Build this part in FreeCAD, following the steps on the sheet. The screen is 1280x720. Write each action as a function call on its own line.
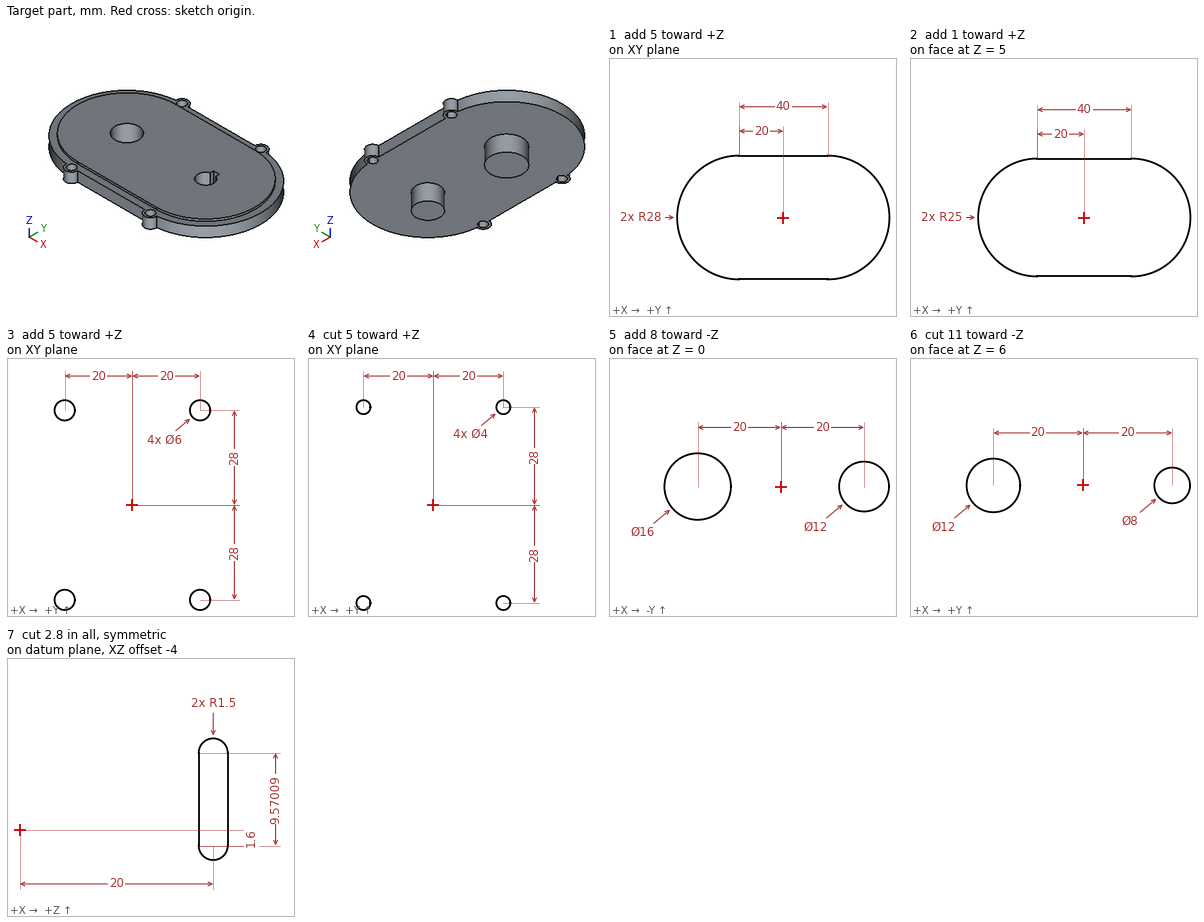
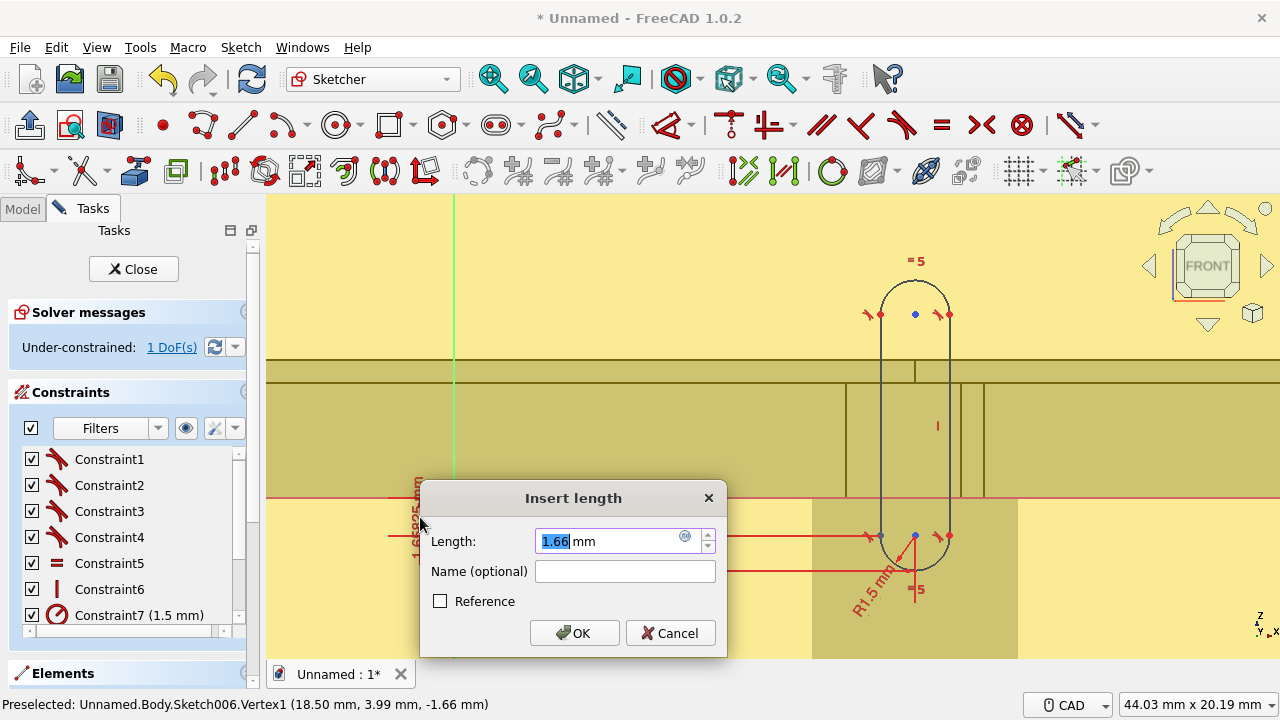
text(1.6)
key(Return)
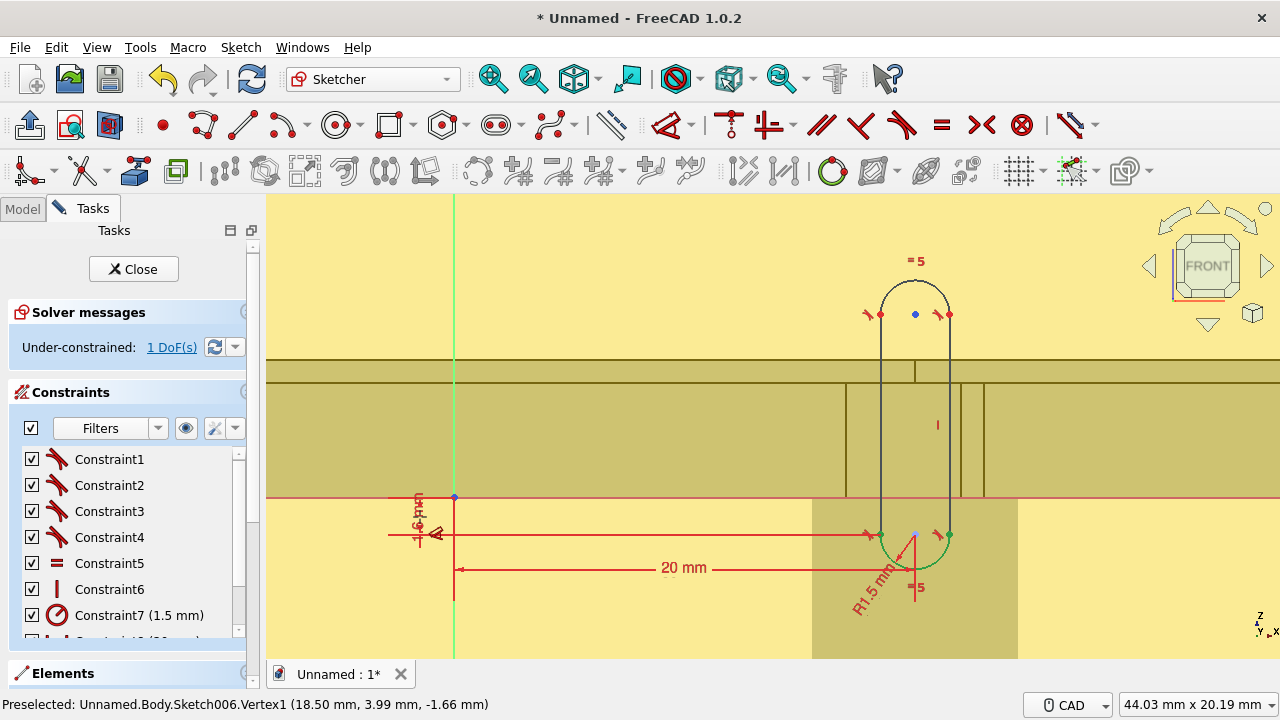
click(881, 469)
click(915, 425)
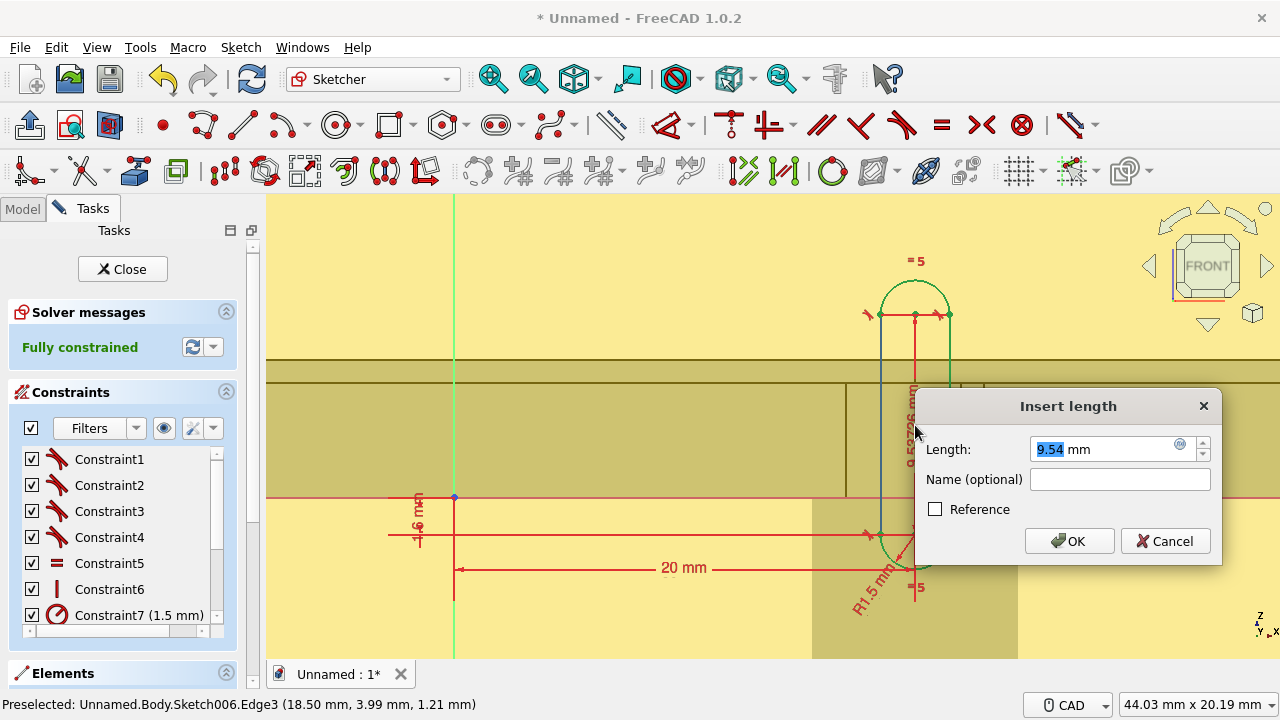
text(9.57009)
key(Return)
key(Escape)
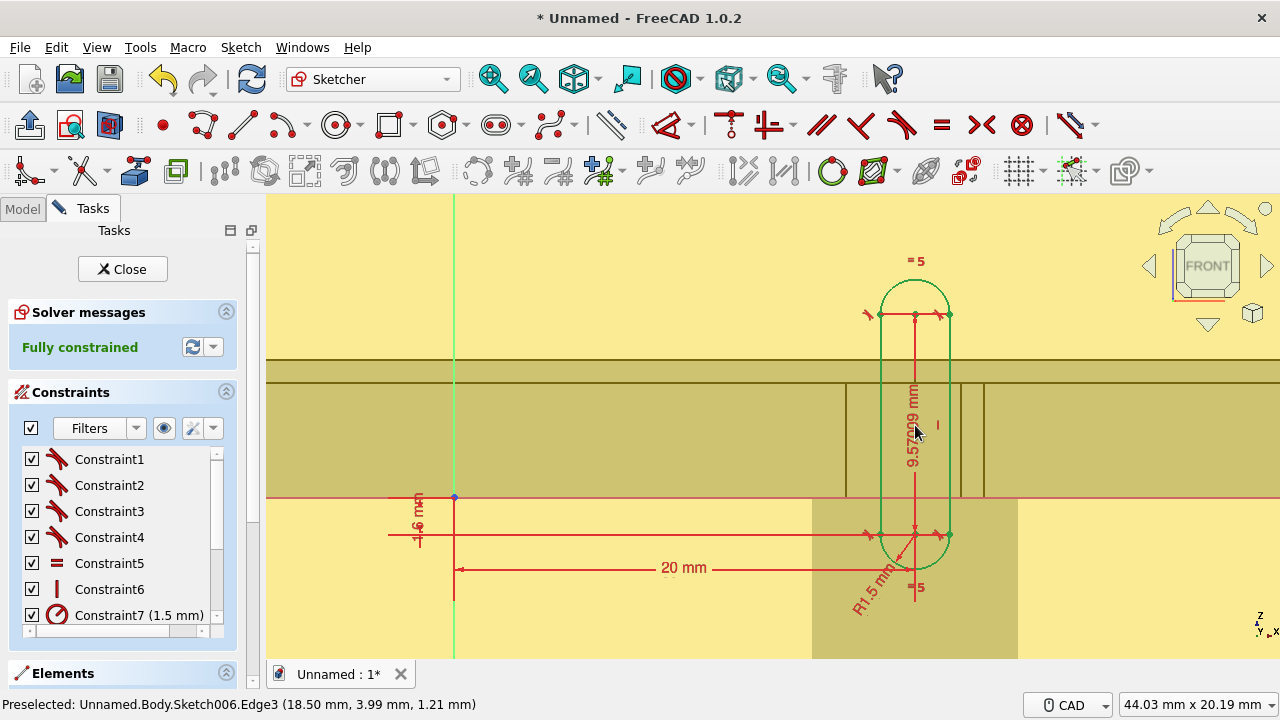
click(123, 269)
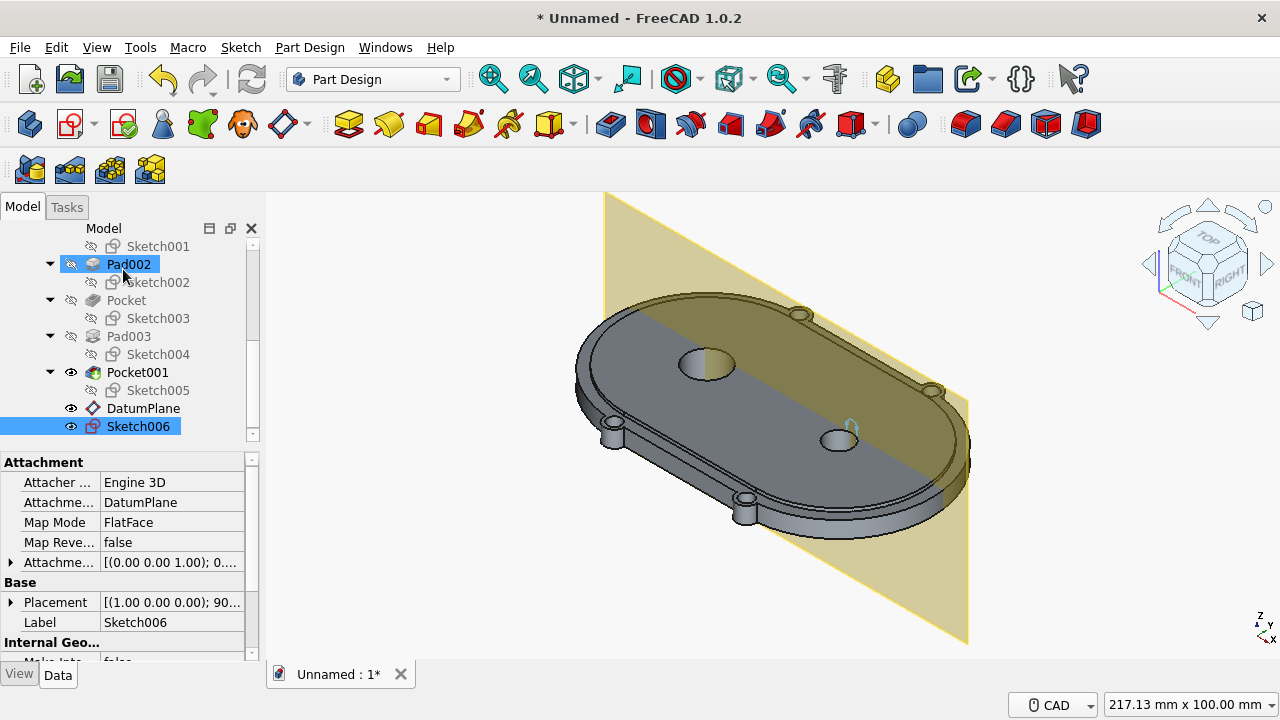
click(612, 124)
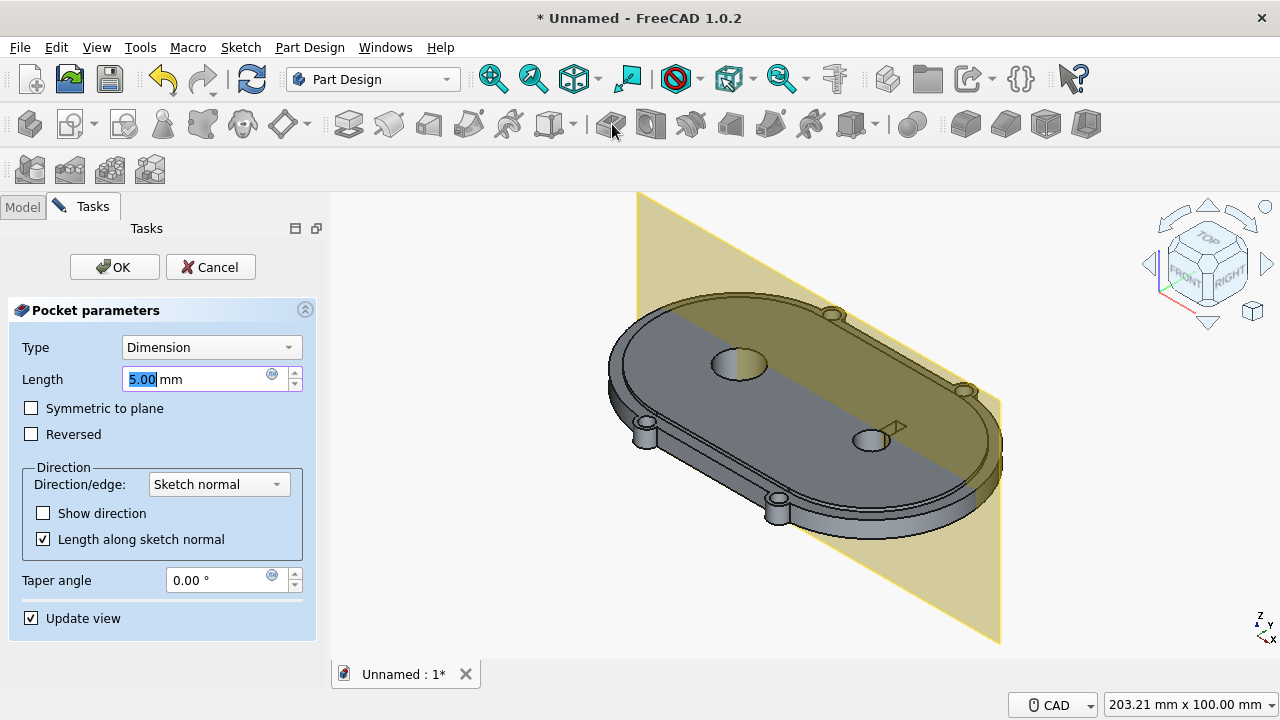
text(2.8)
key(Tab)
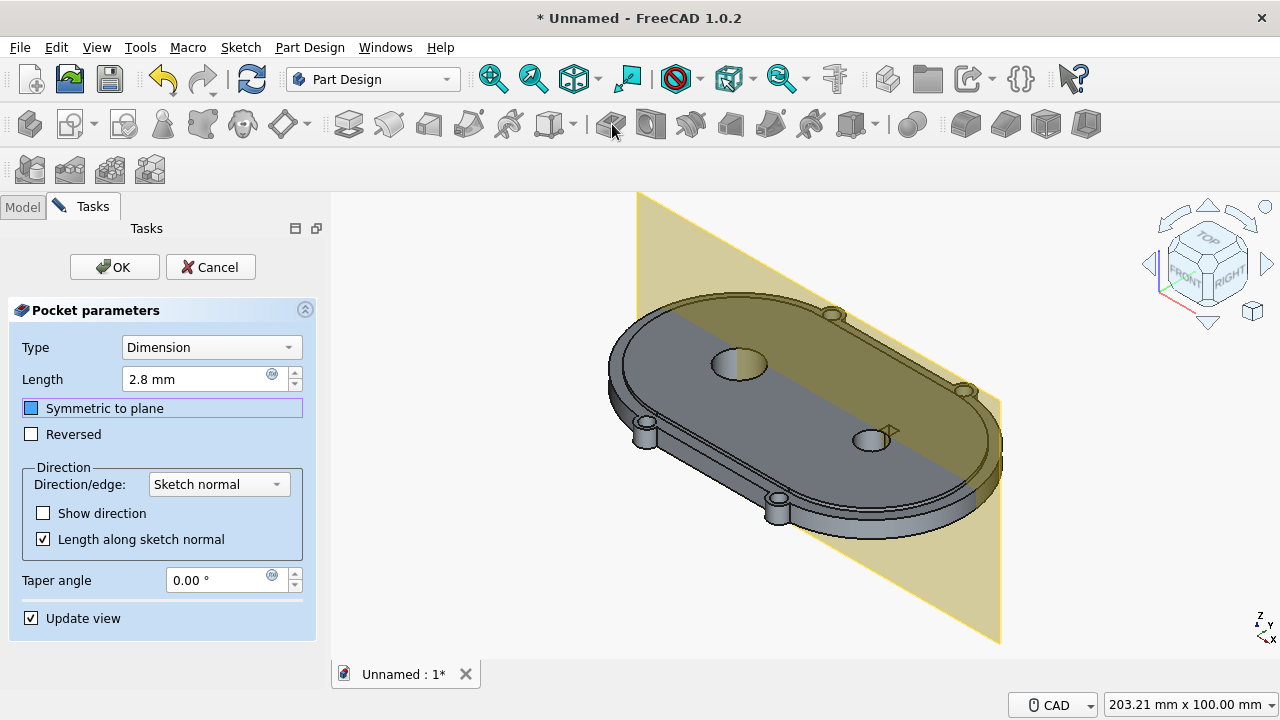
click(30, 408)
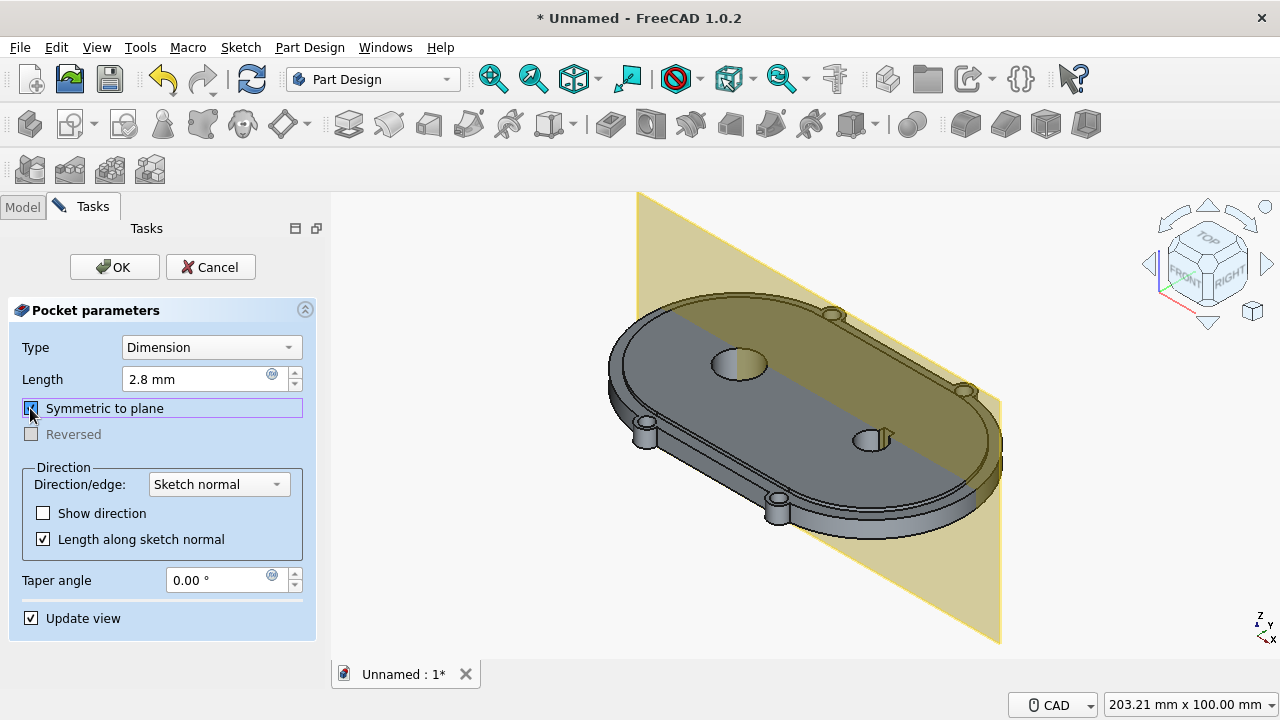
click(115, 267)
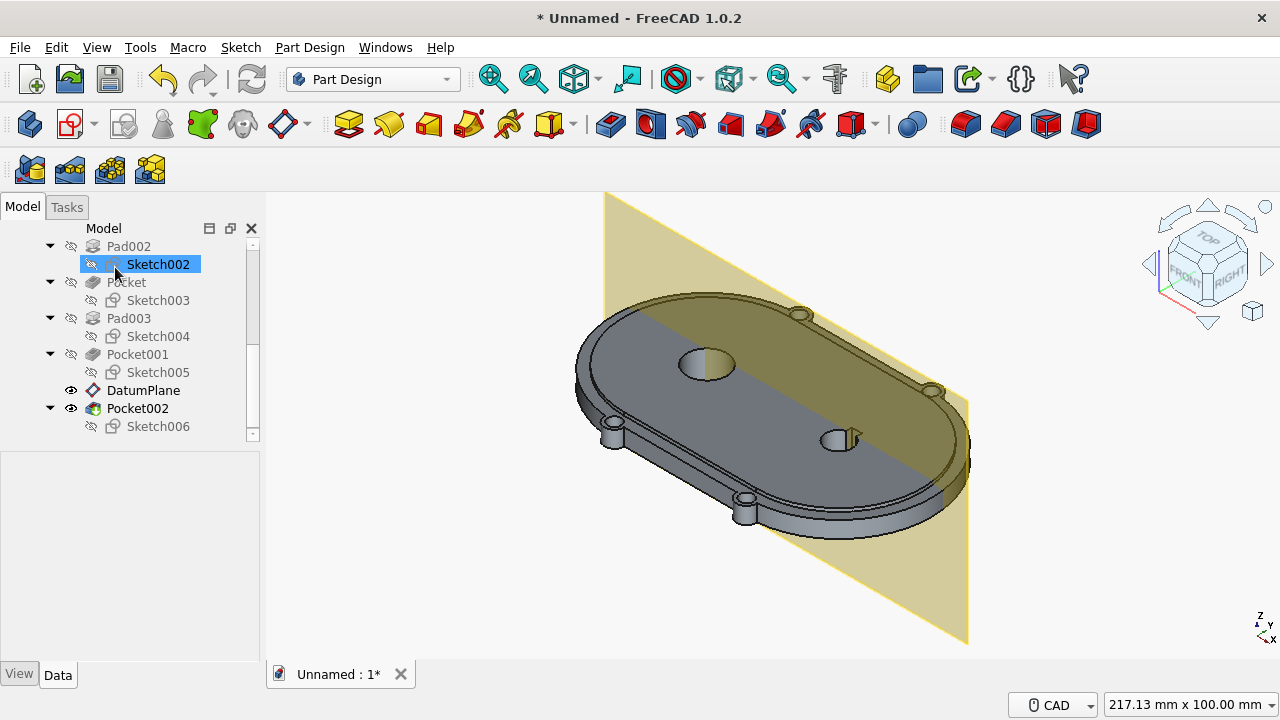
click(116, 390)
key(space)